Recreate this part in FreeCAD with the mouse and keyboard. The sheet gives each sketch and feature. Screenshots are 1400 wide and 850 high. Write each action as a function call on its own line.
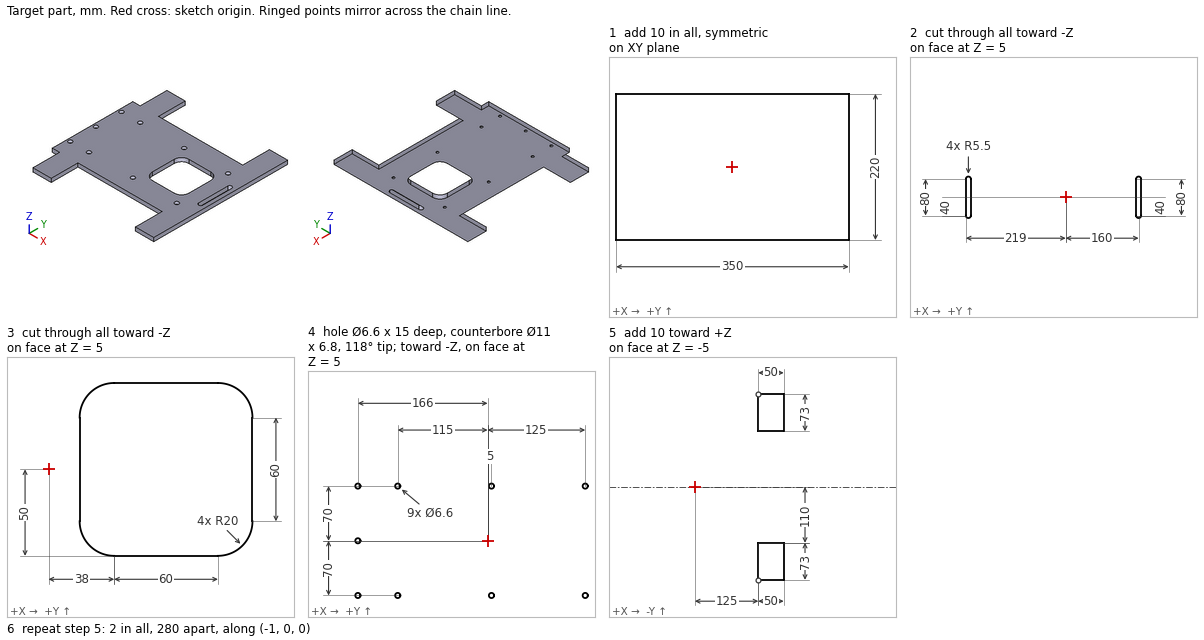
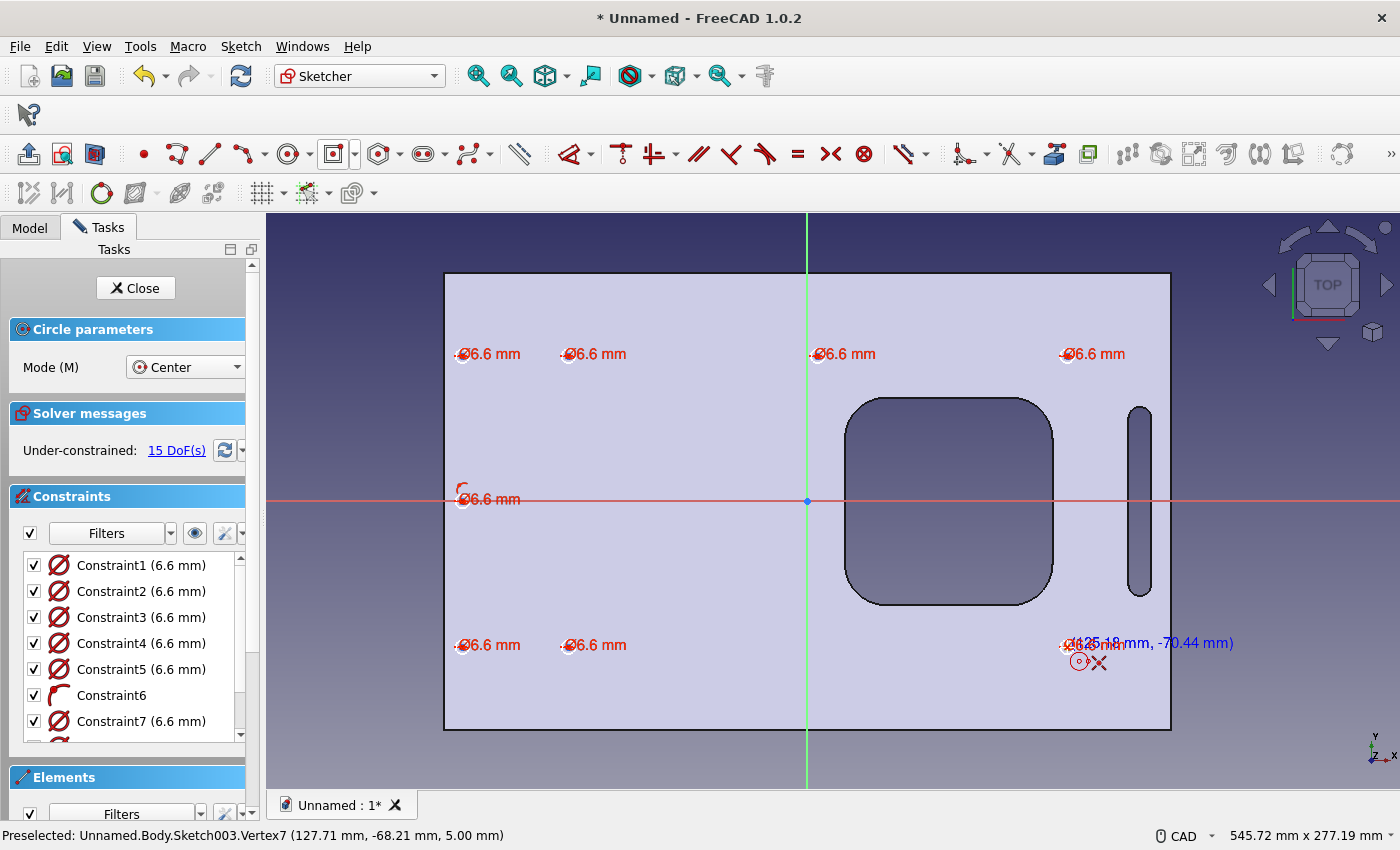
scroll(818, 647, up, 6)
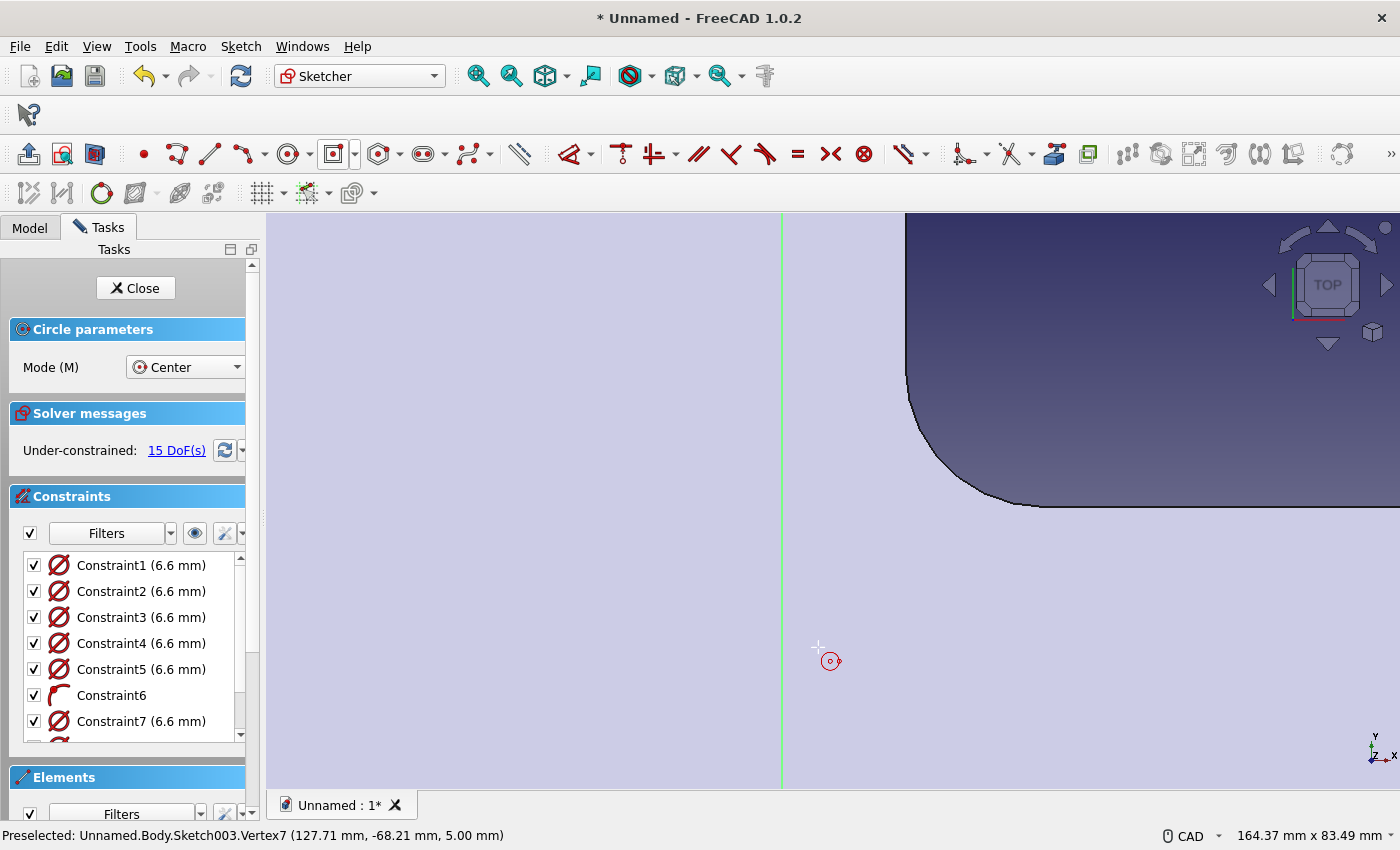
click(816, 645)
move(832, 629)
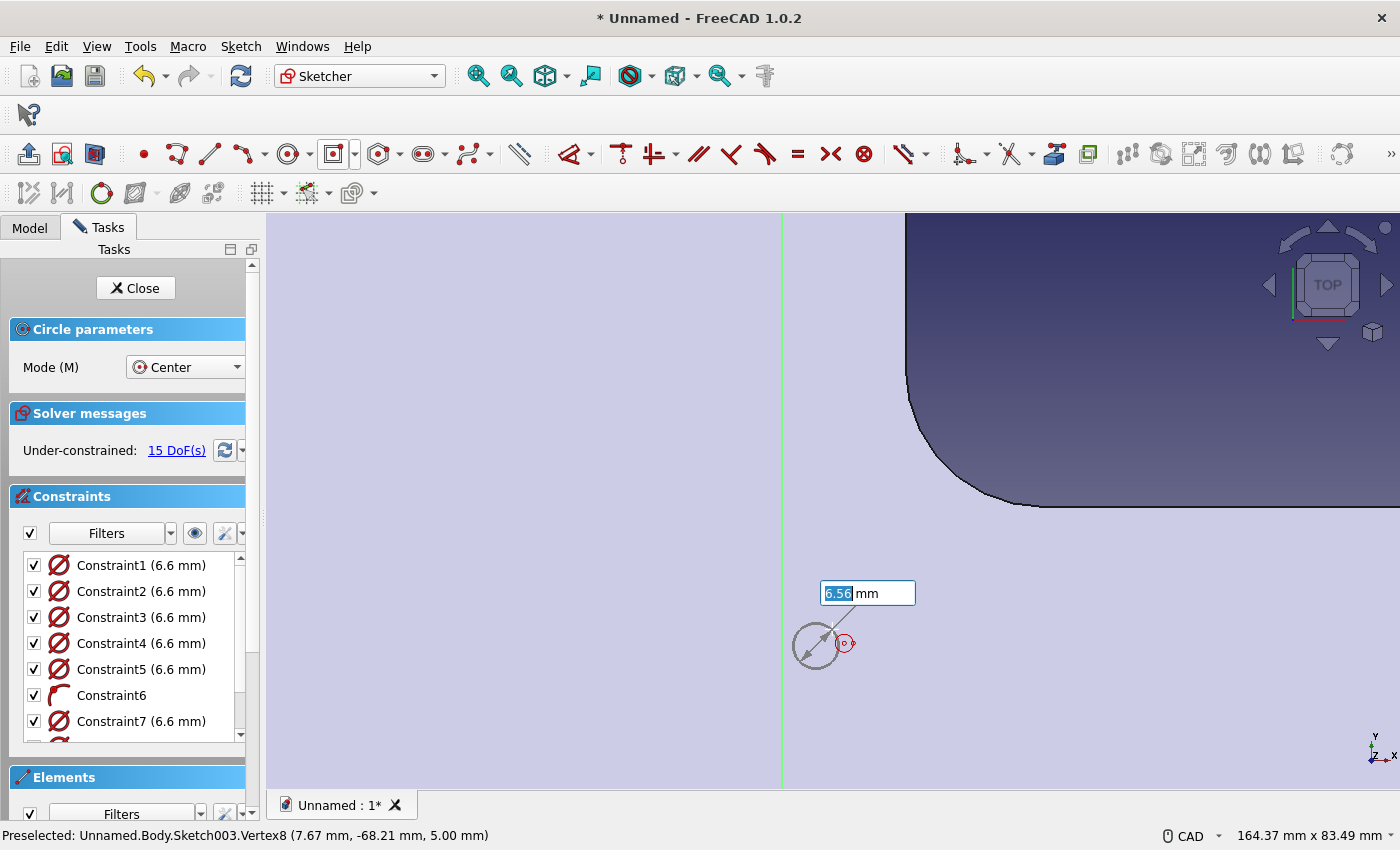
text(6.6)
key(Return)
key(Escape)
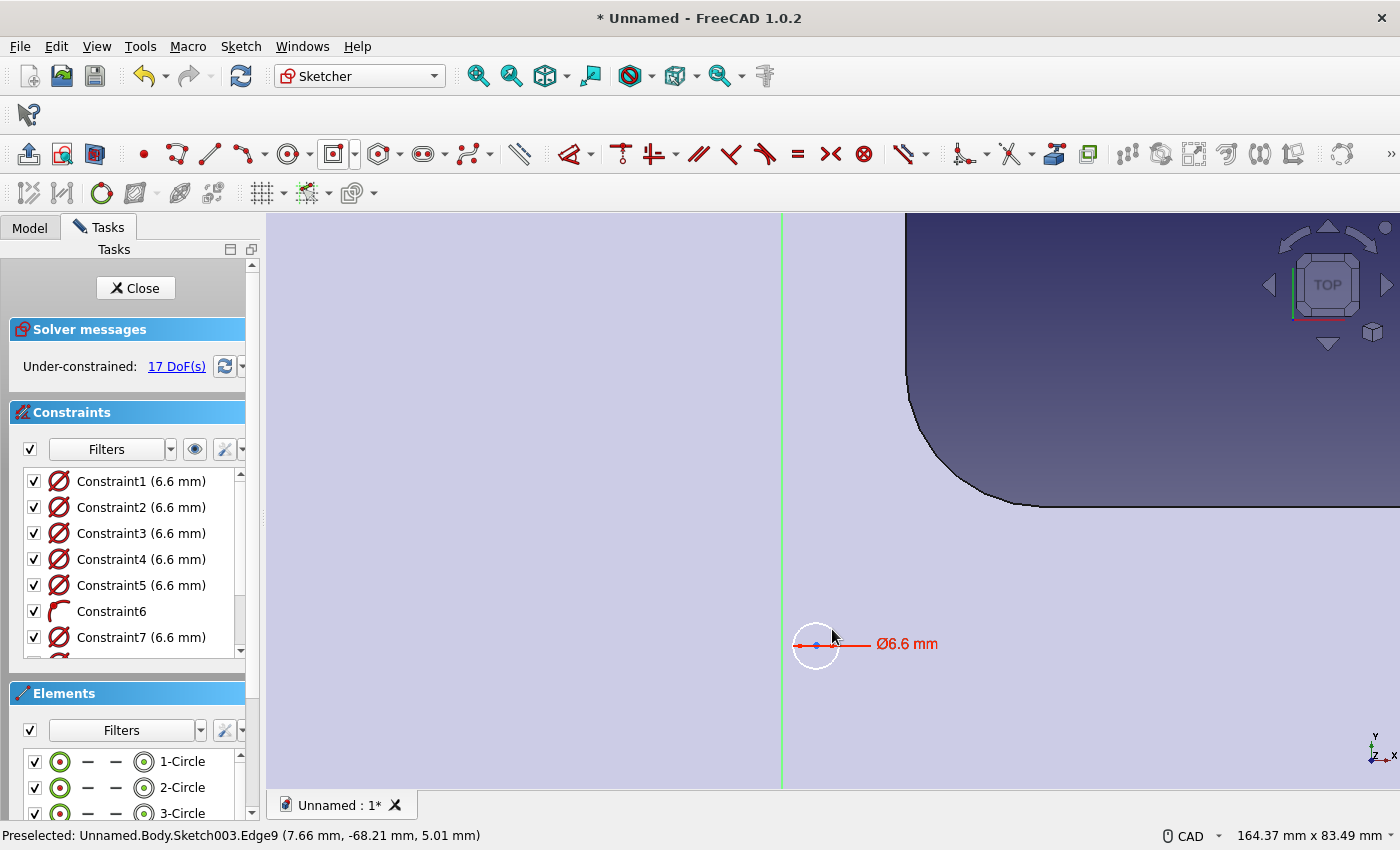
scroll(818, 647, down, 6)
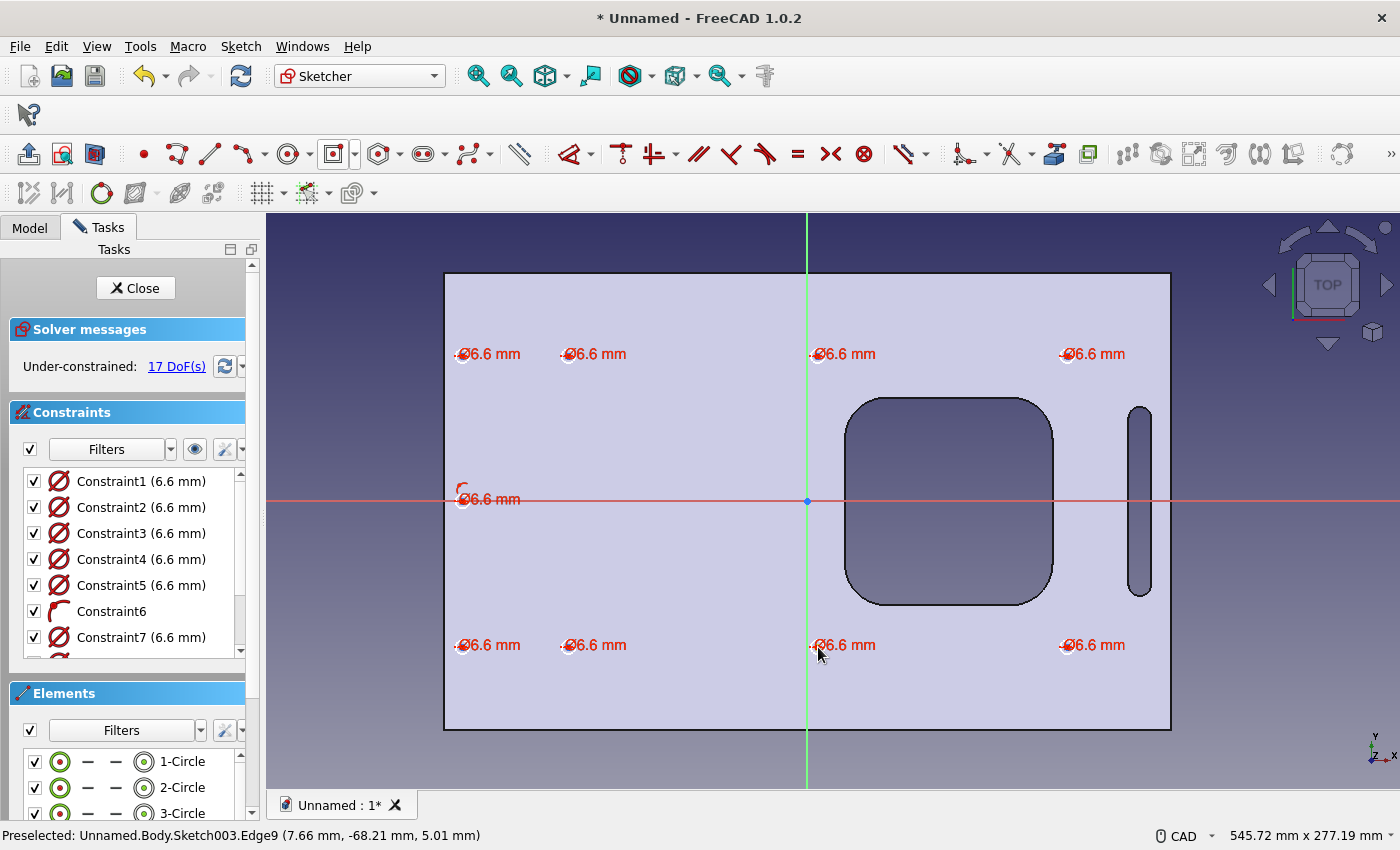
click(568, 356)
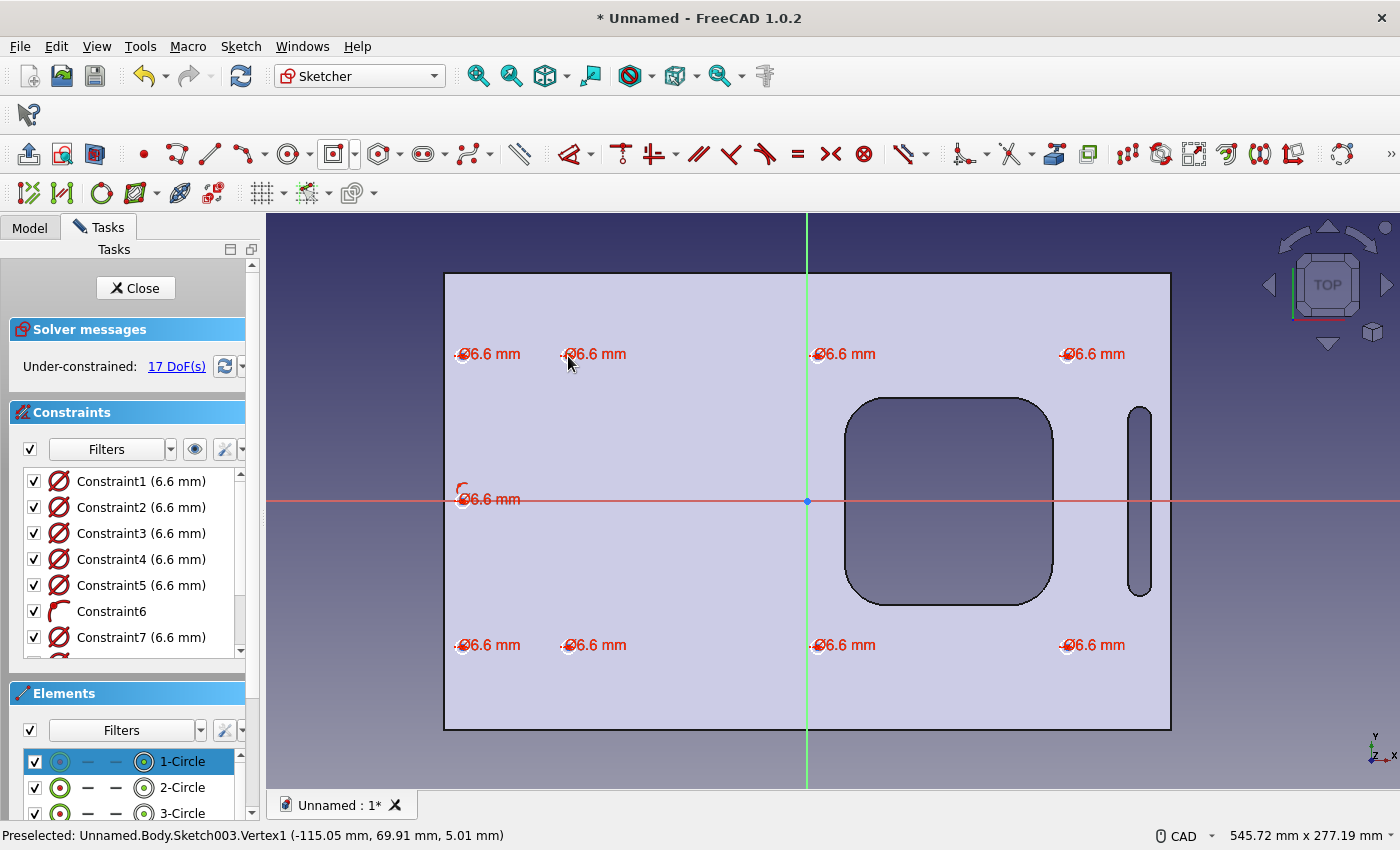
click(568, 647)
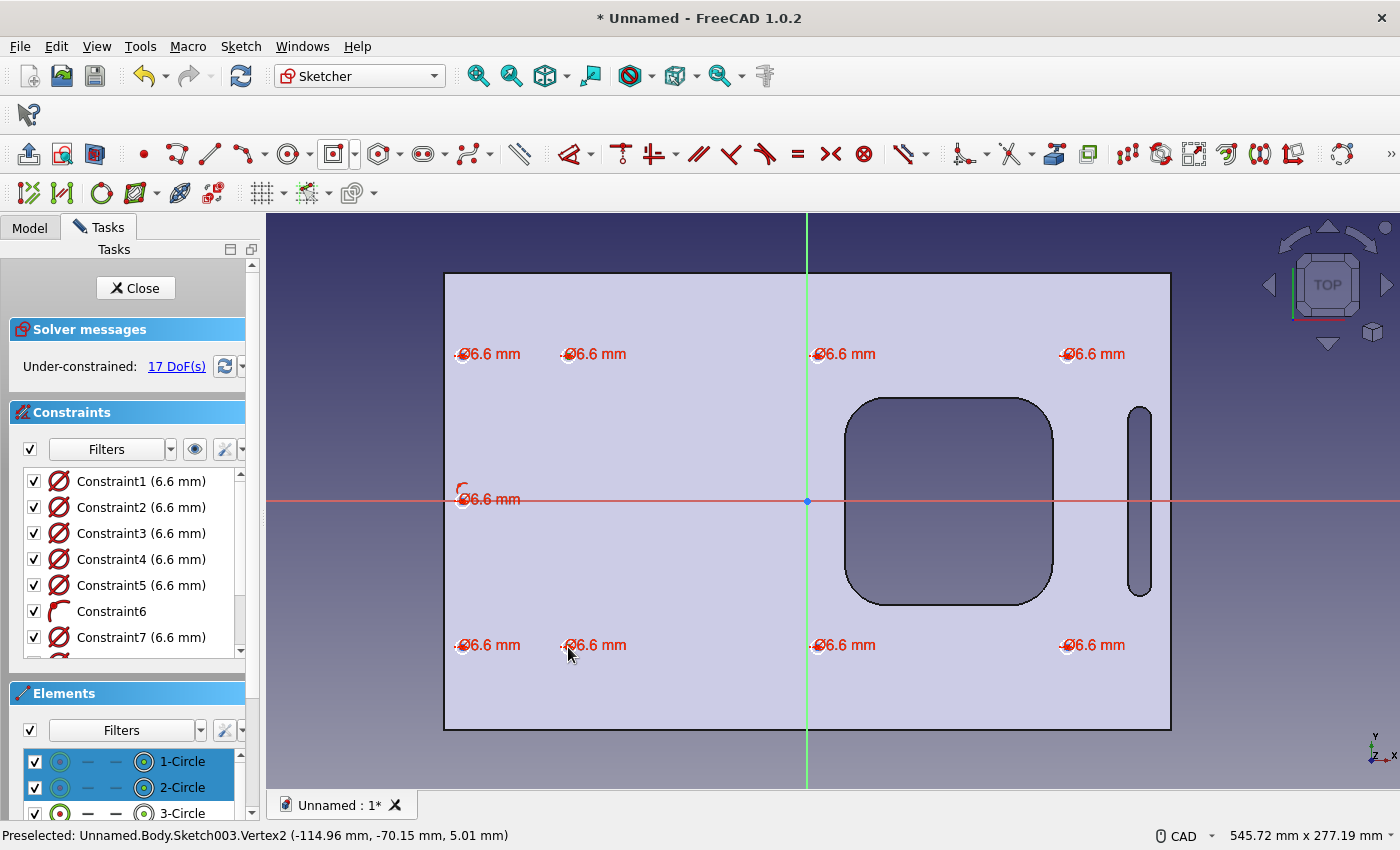
click(676, 154)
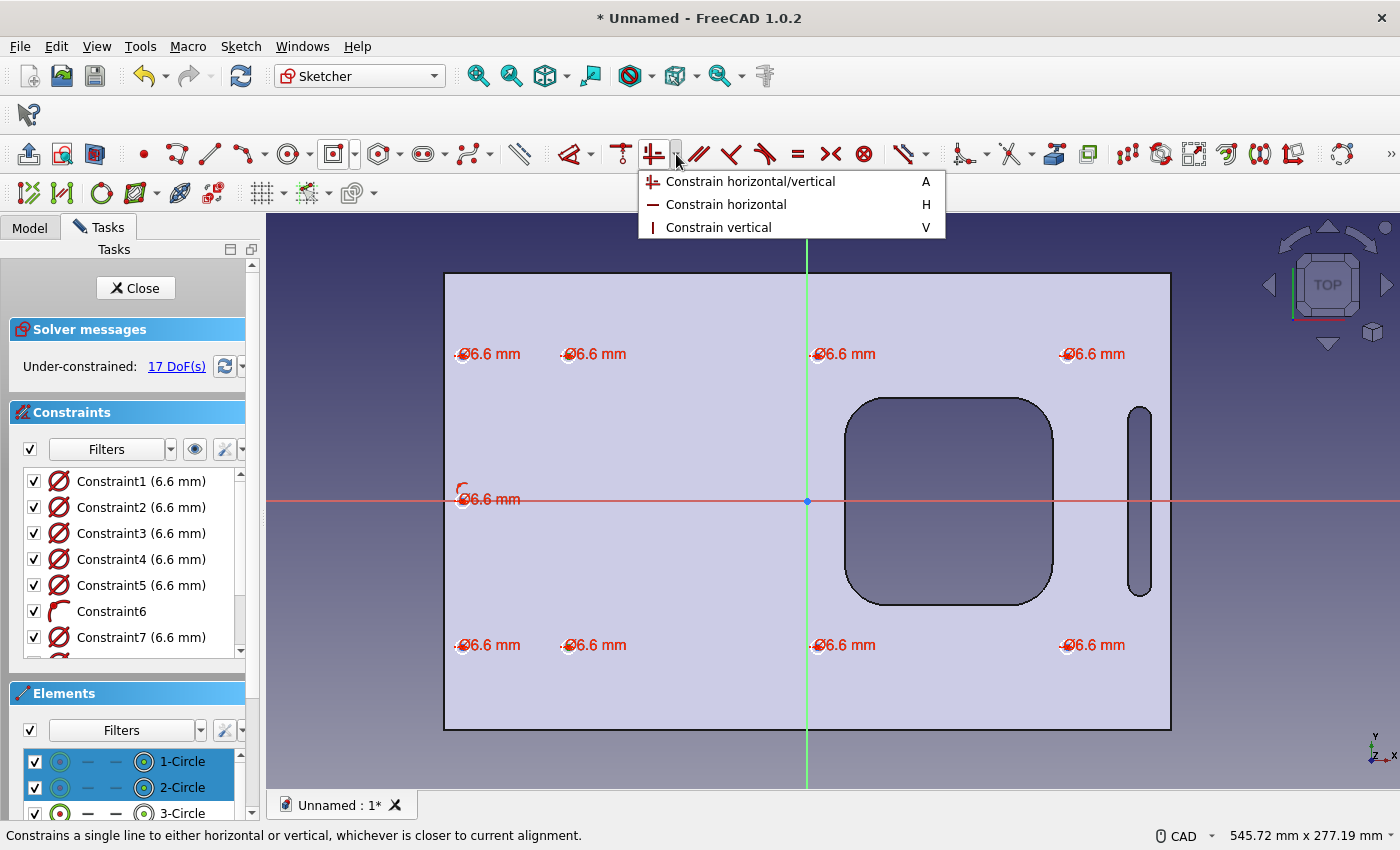
click(792, 228)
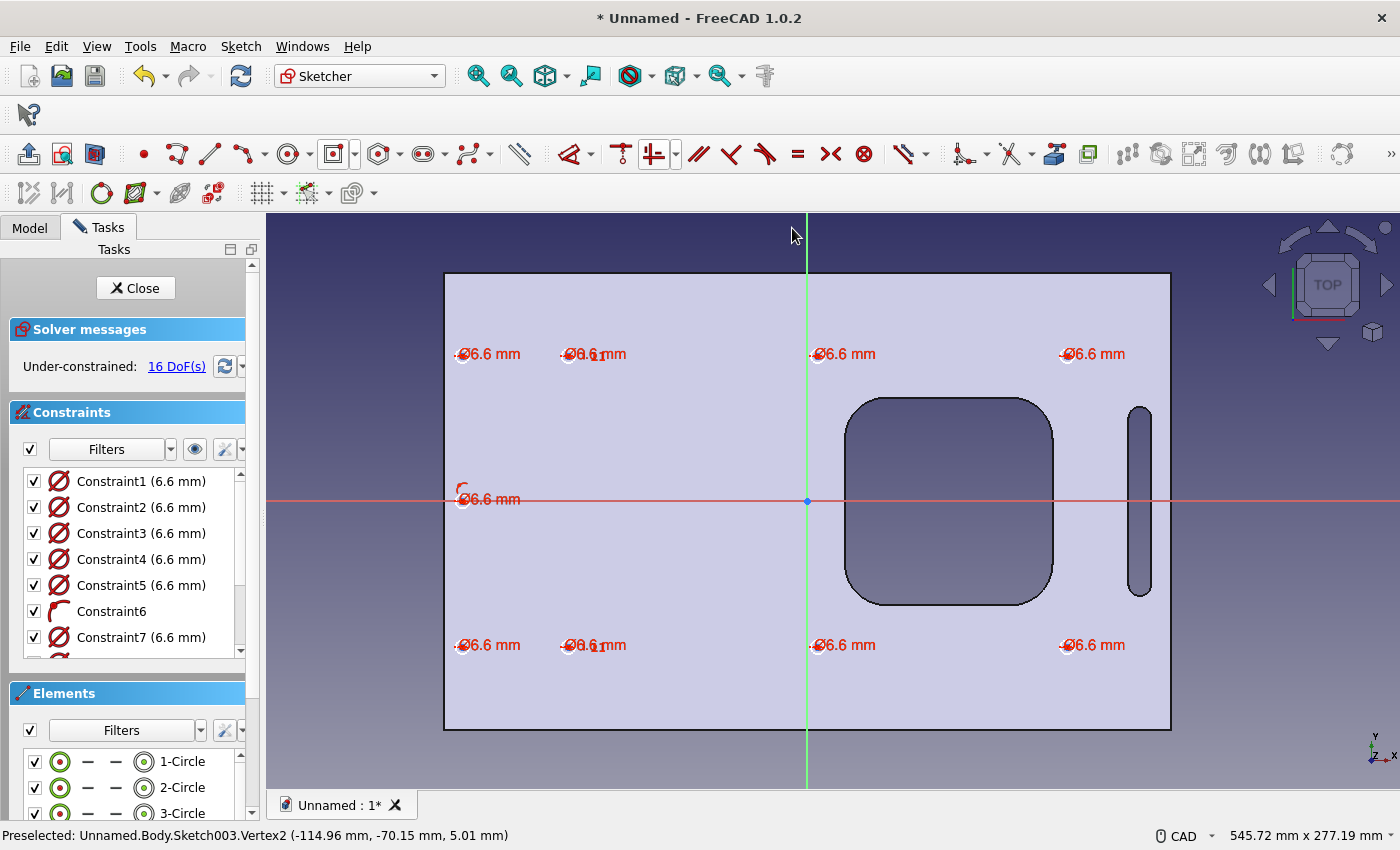
click(568, 356)